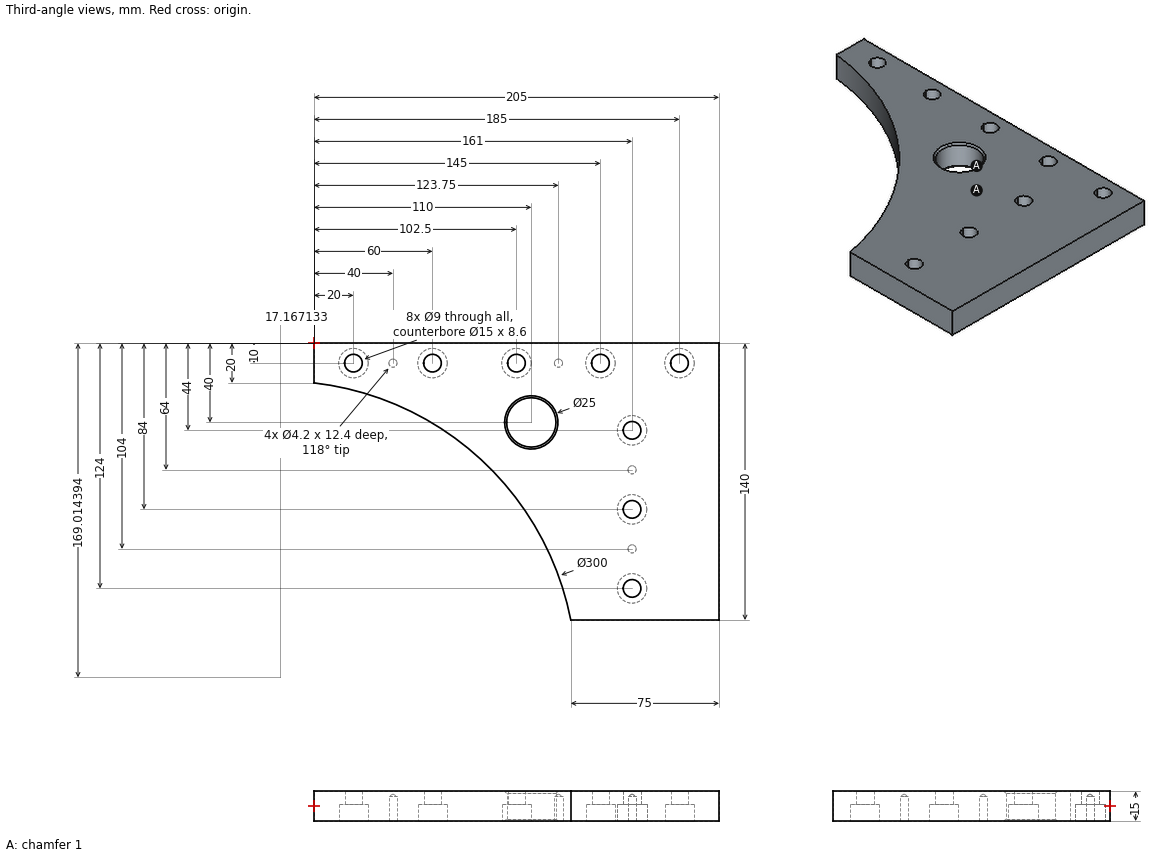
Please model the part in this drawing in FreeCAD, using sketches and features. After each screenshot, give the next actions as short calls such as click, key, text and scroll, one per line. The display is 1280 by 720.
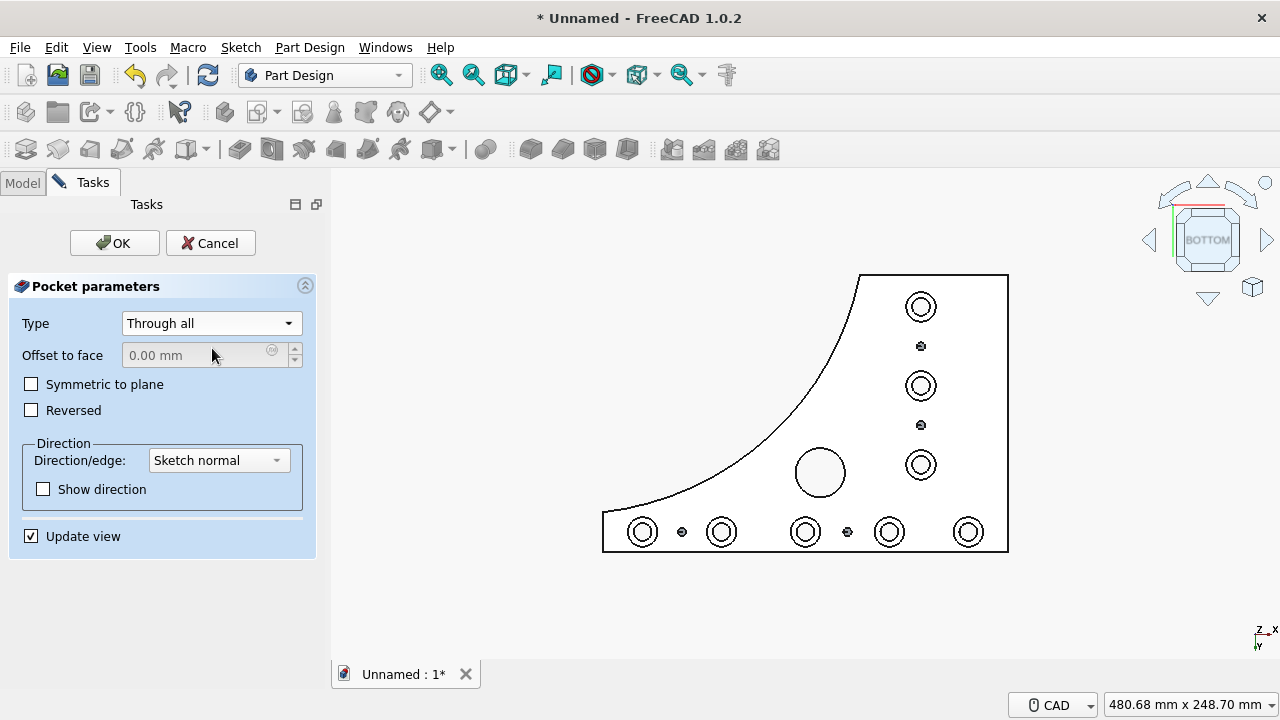
click(115, 243)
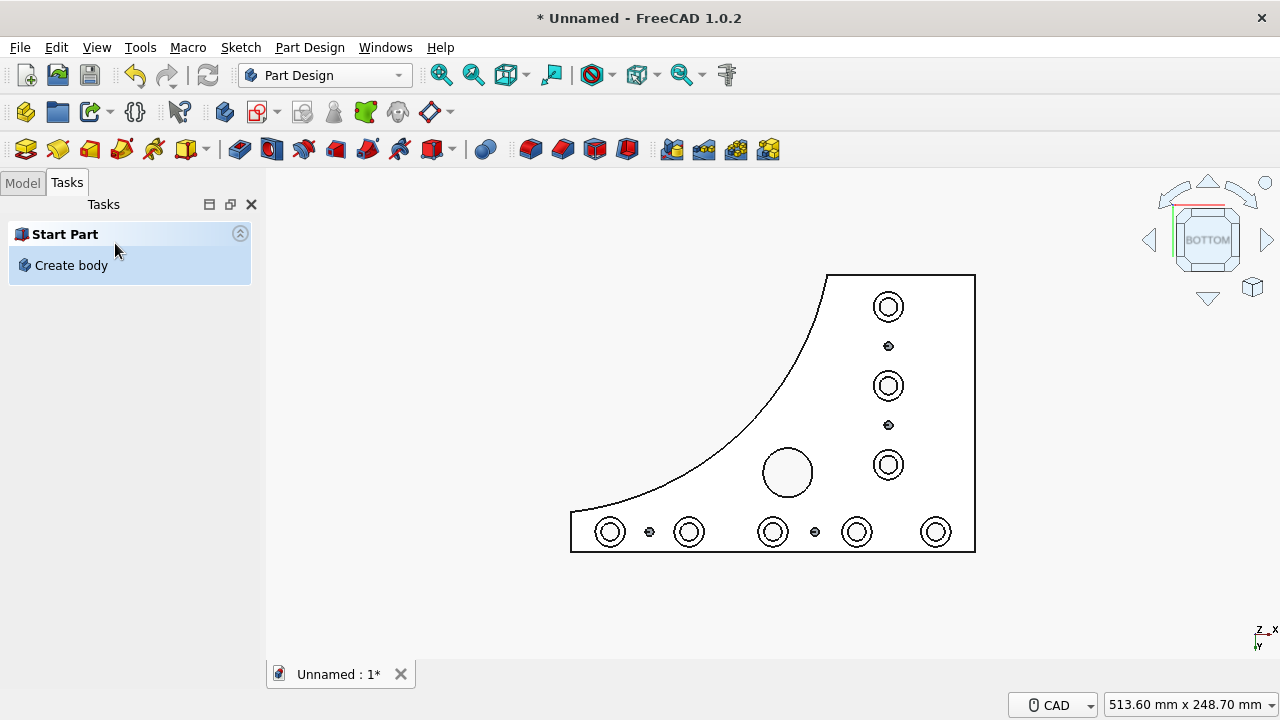
click(768, 457)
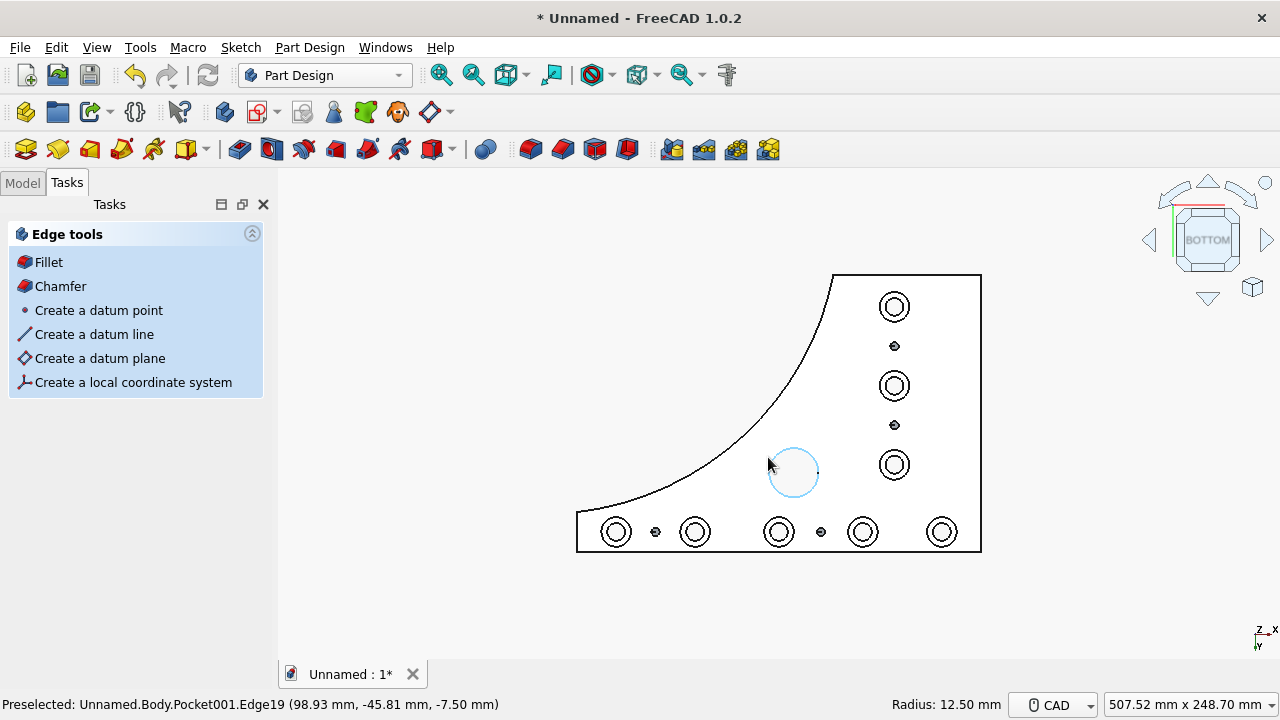
key(0)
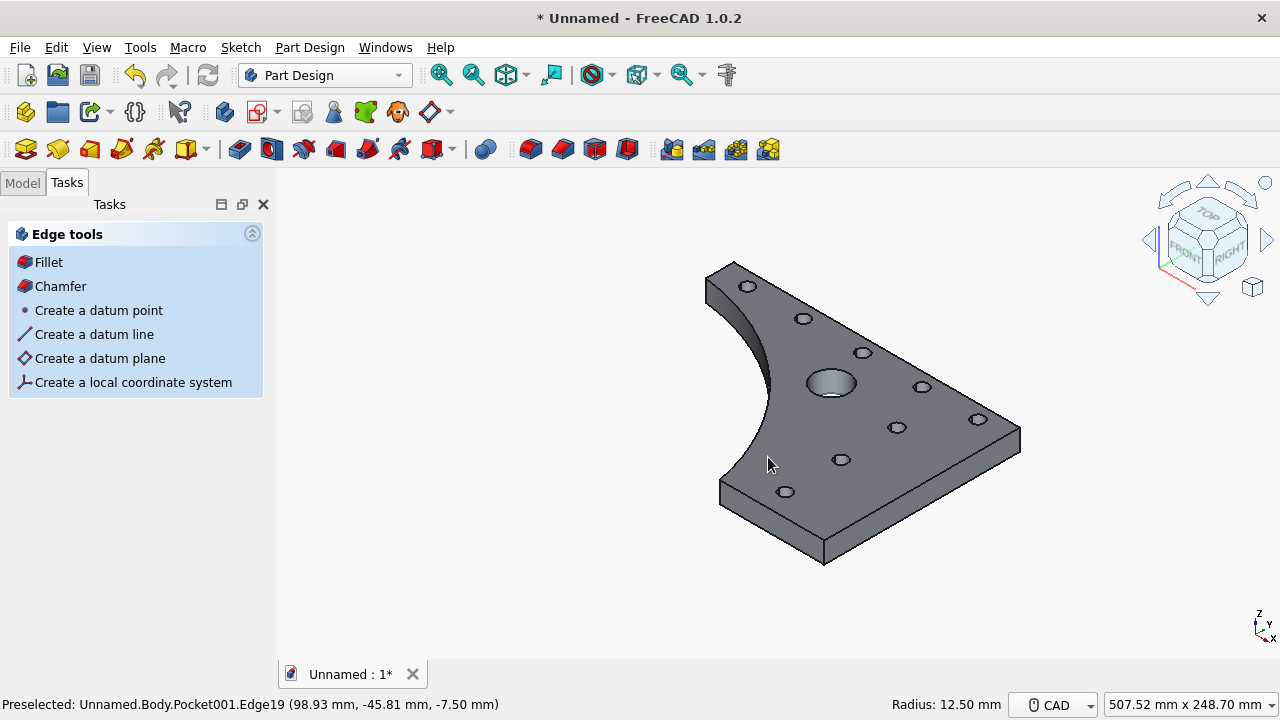
click(814, 372, ctrl)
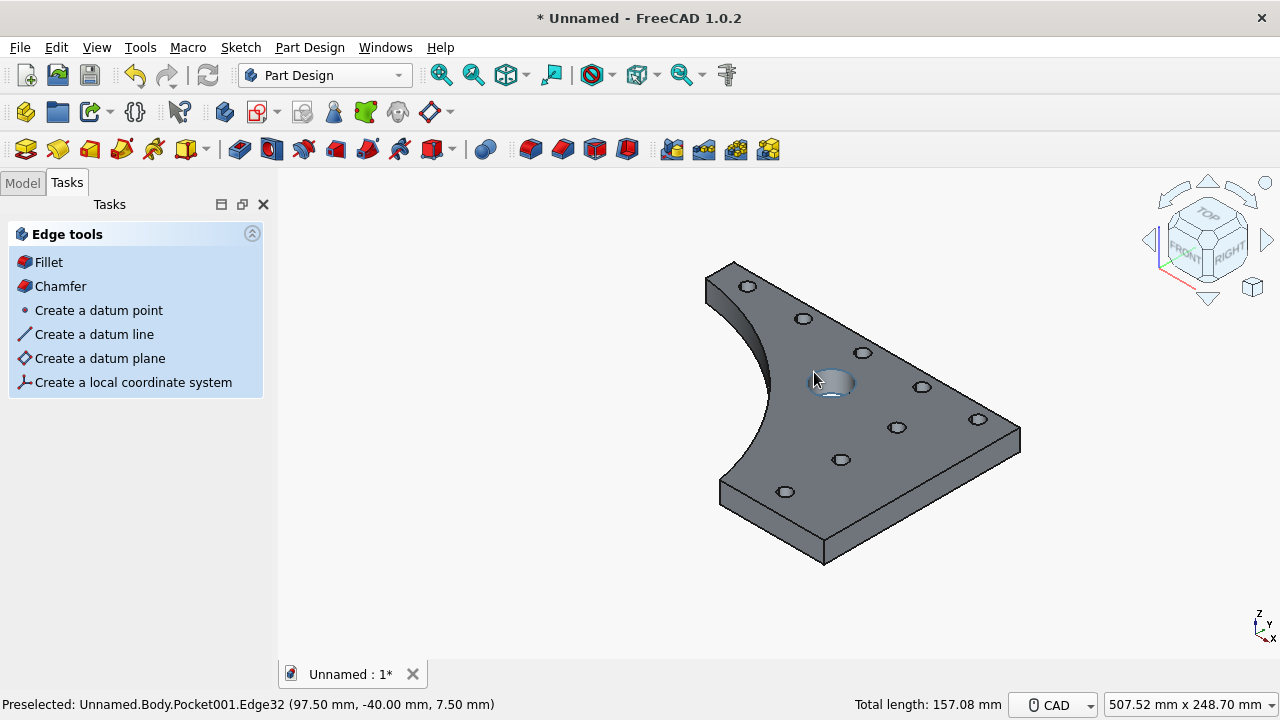
click(564, 150)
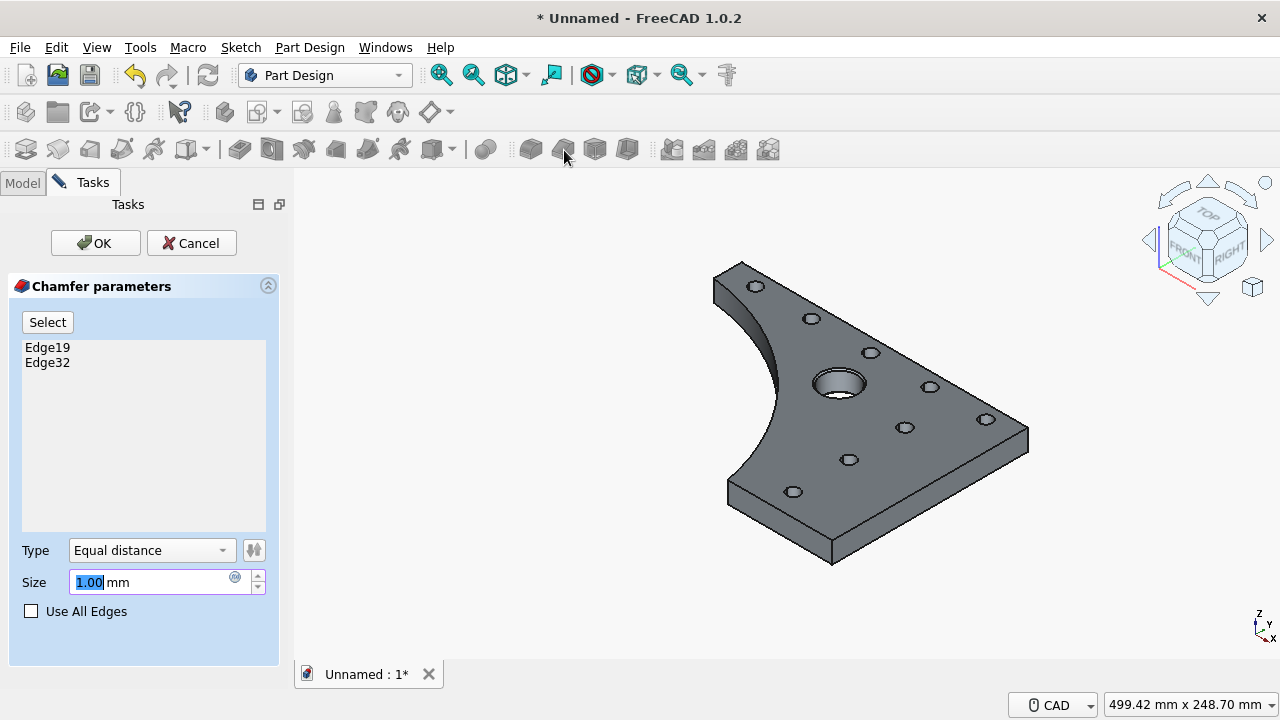
text(1)
key(Tab)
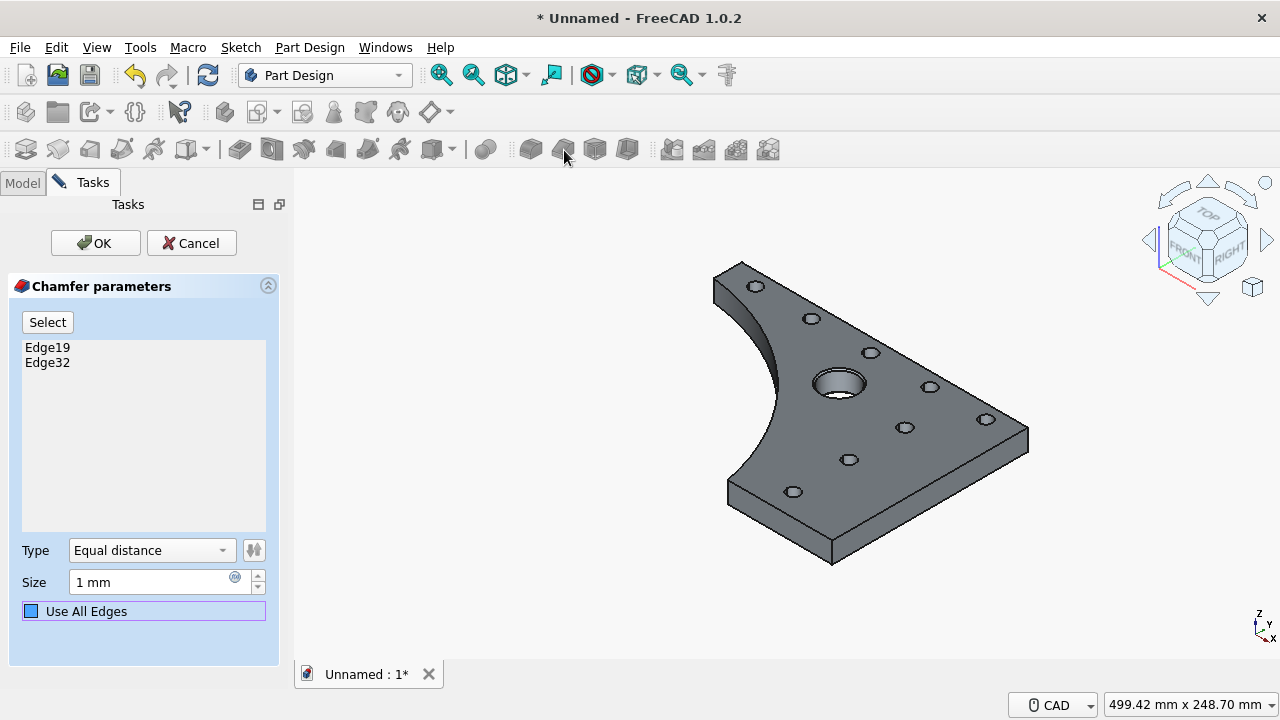
click(96, 243)